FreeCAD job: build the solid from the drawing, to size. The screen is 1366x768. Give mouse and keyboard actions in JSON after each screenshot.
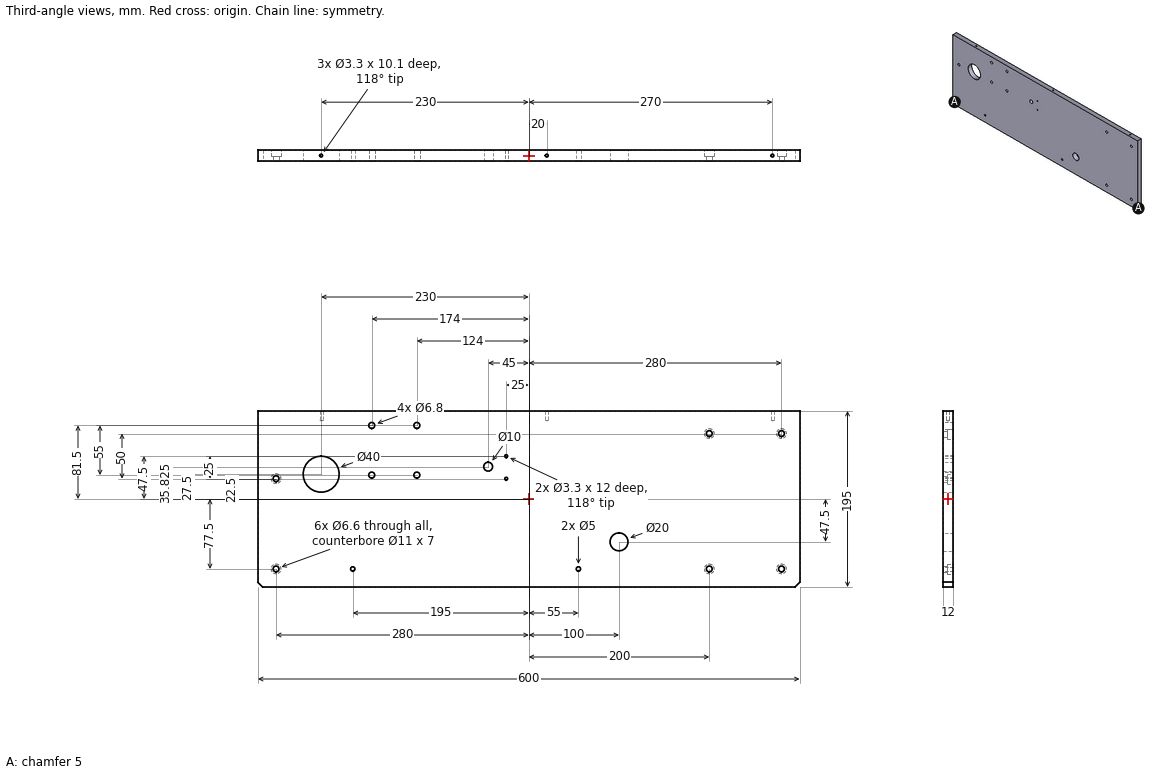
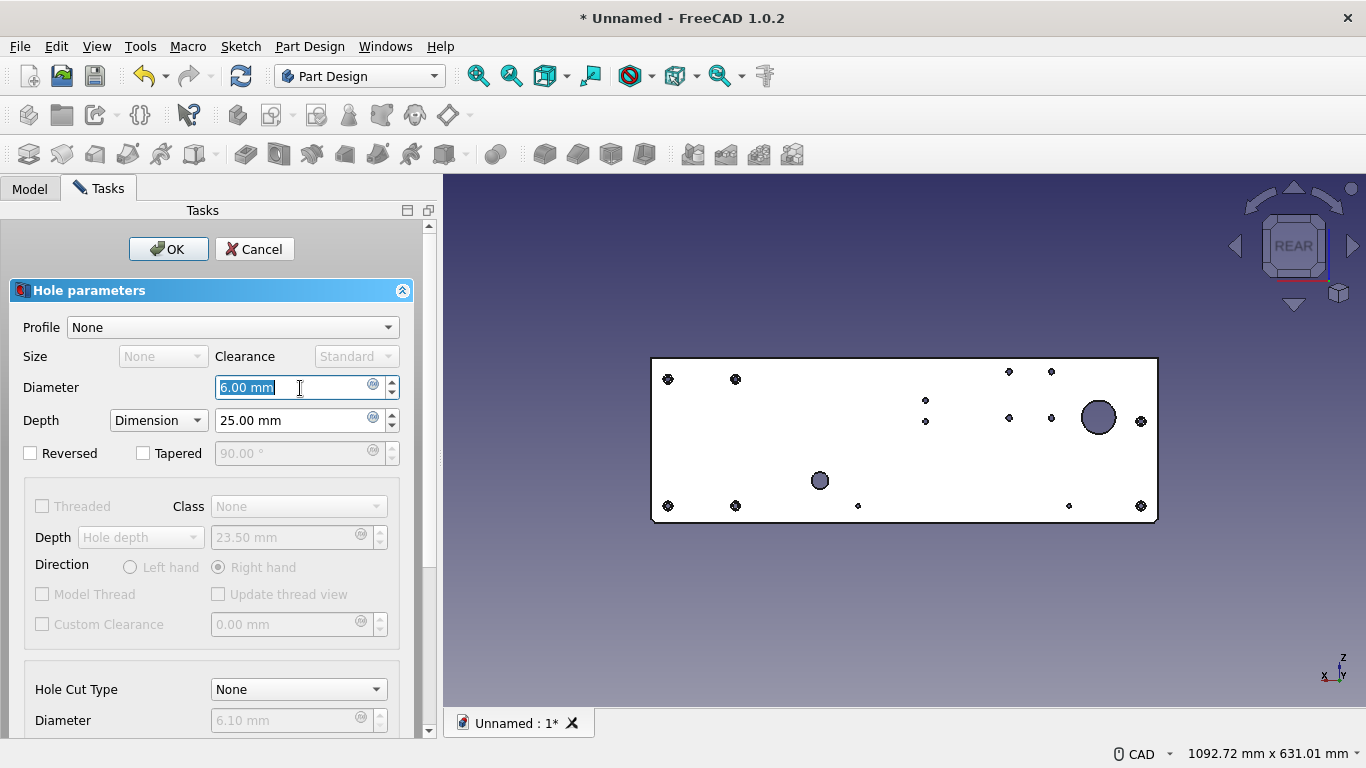
{"action": "type", "text": "3.3"}
{"action": "key", "text": "Tab"}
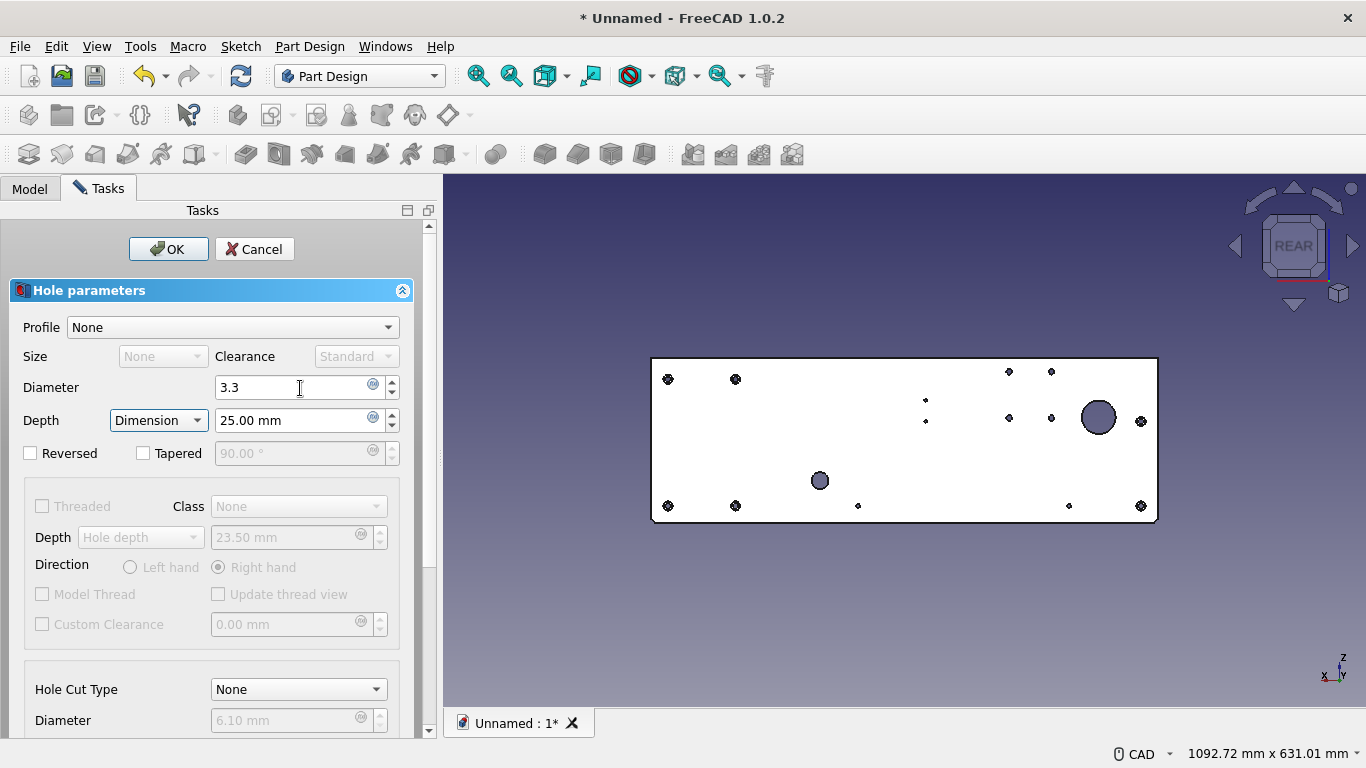
{"action": "triple_click", "coordinate": [300, 420]}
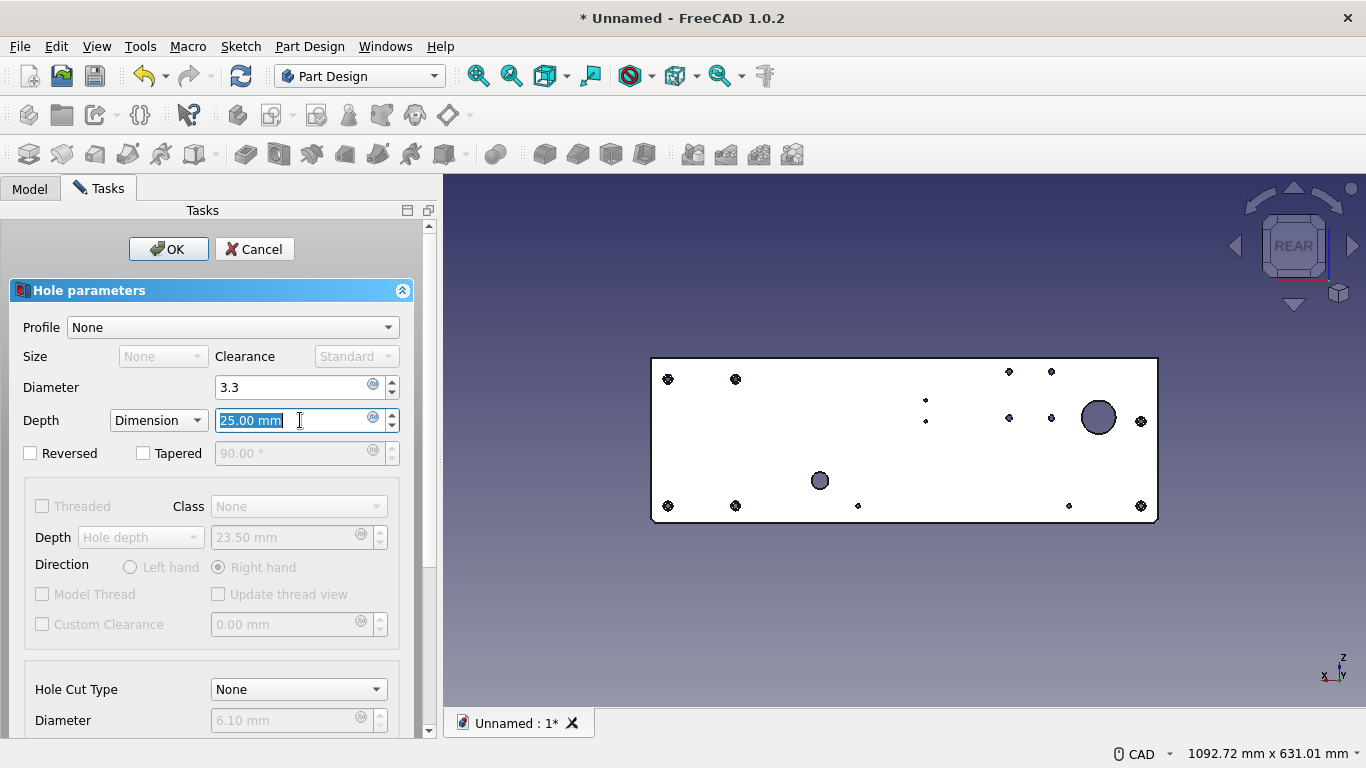
{"action": "type", "text": "12"}
{"action": "key", "text": "Tab"}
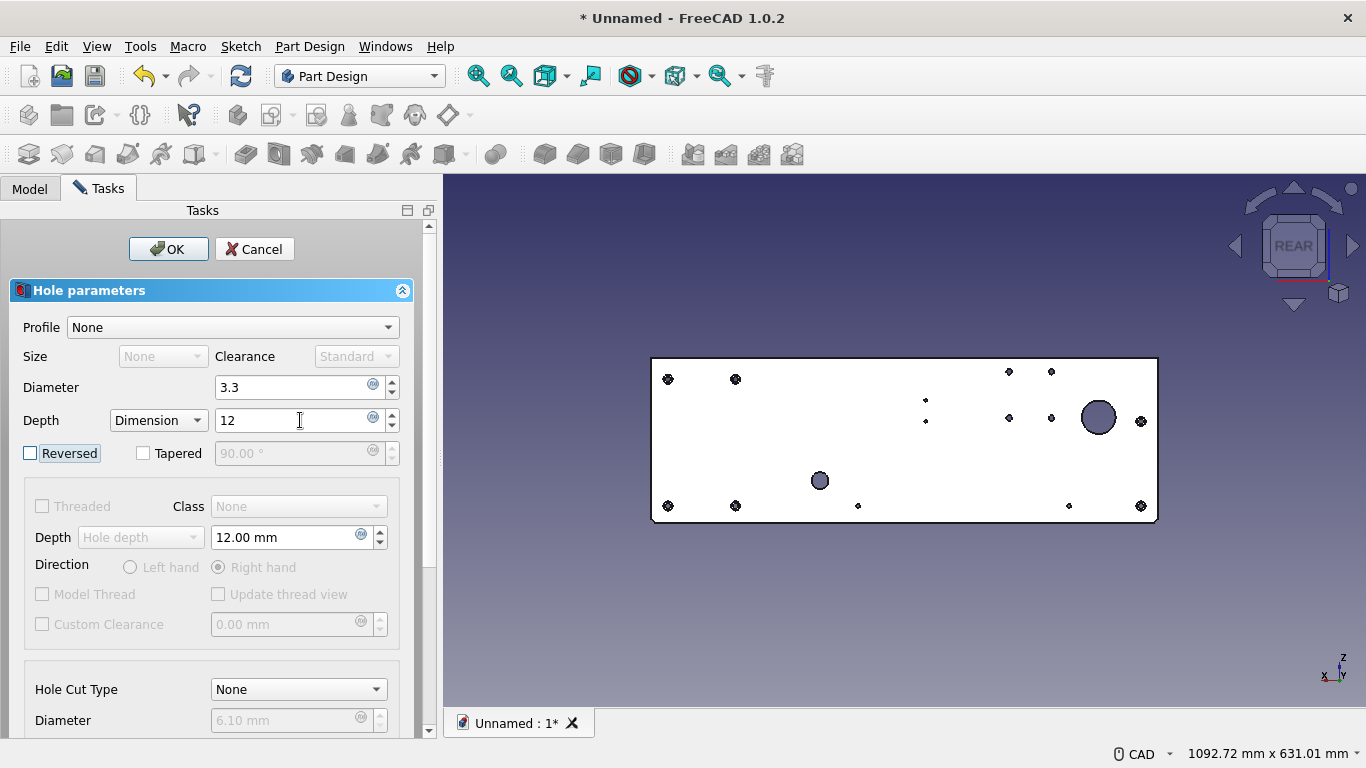
{"action": "left_click", "coordinate": [169, 249]}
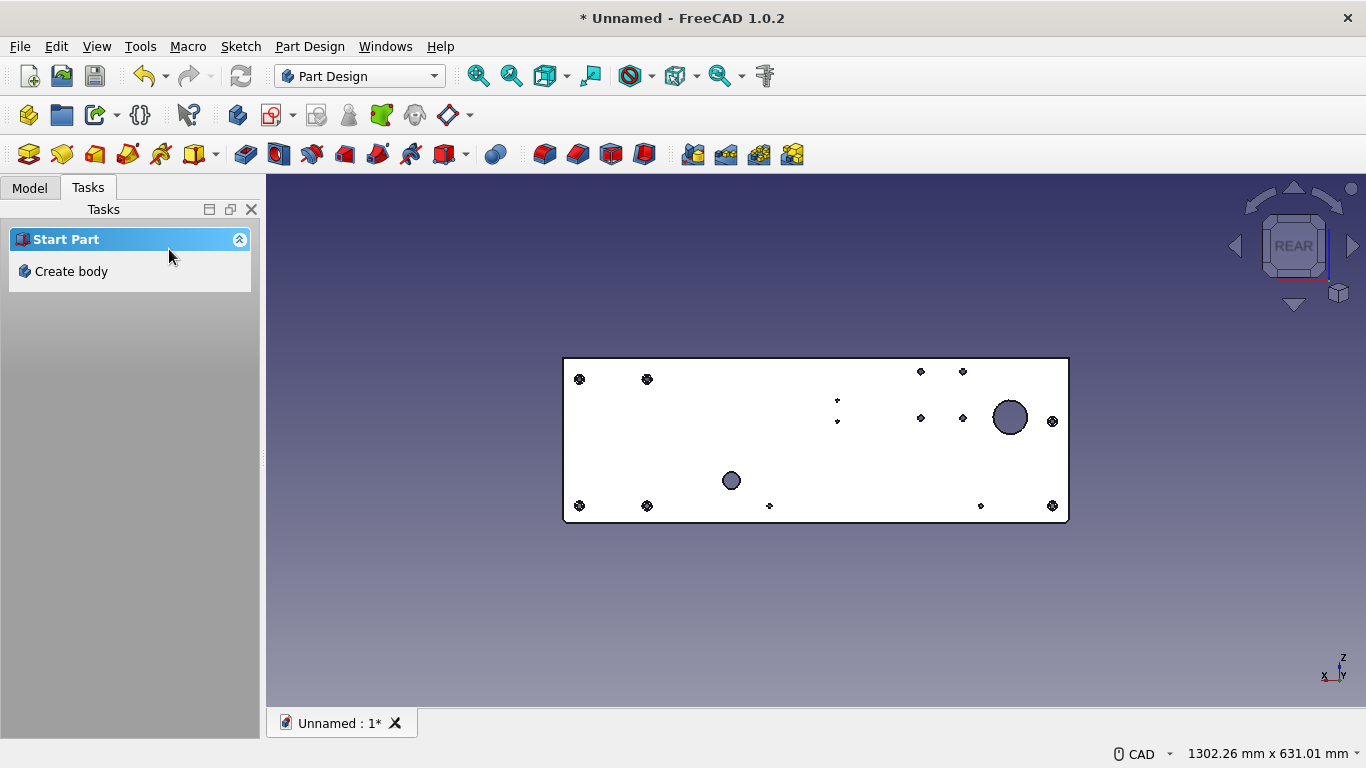
{"action": "left_click", "coordinate": [671, 439]}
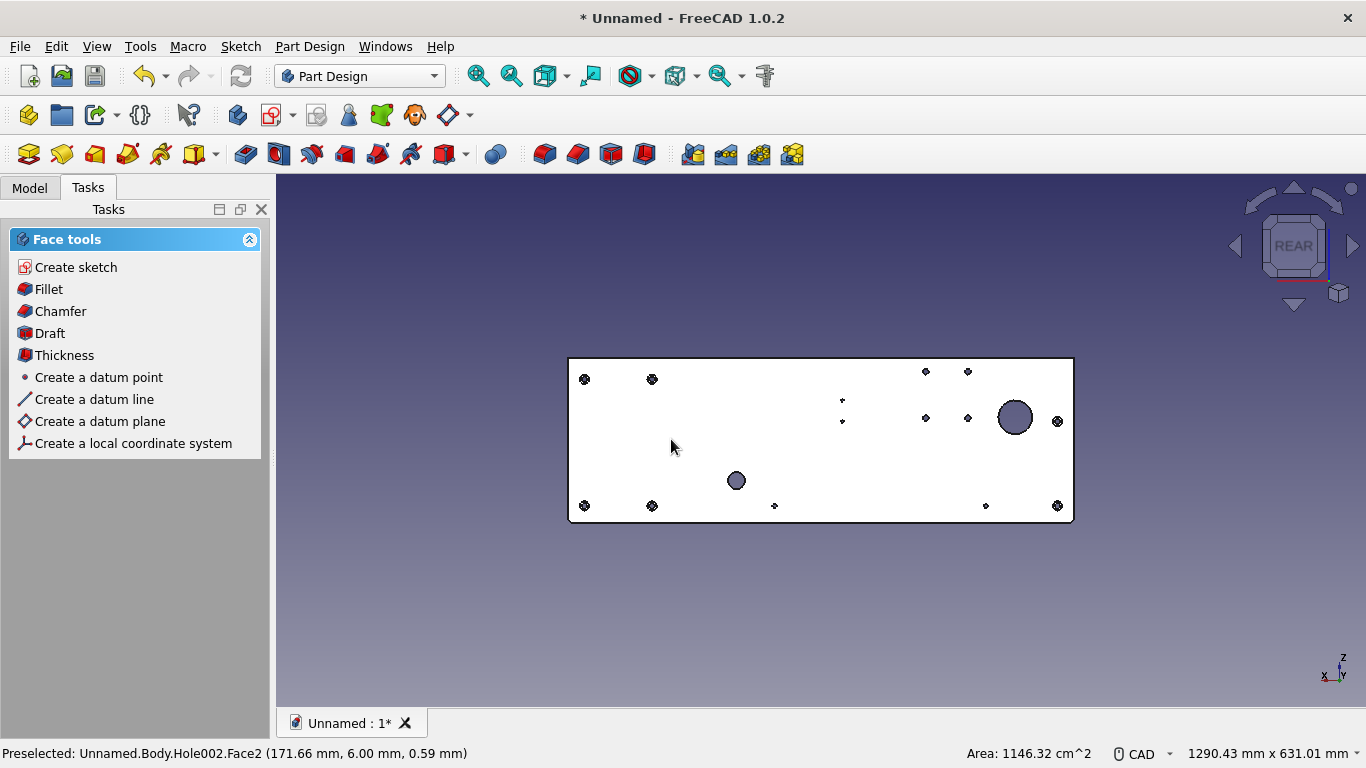
{"action": "left_click", "coordinate": [270, 116]}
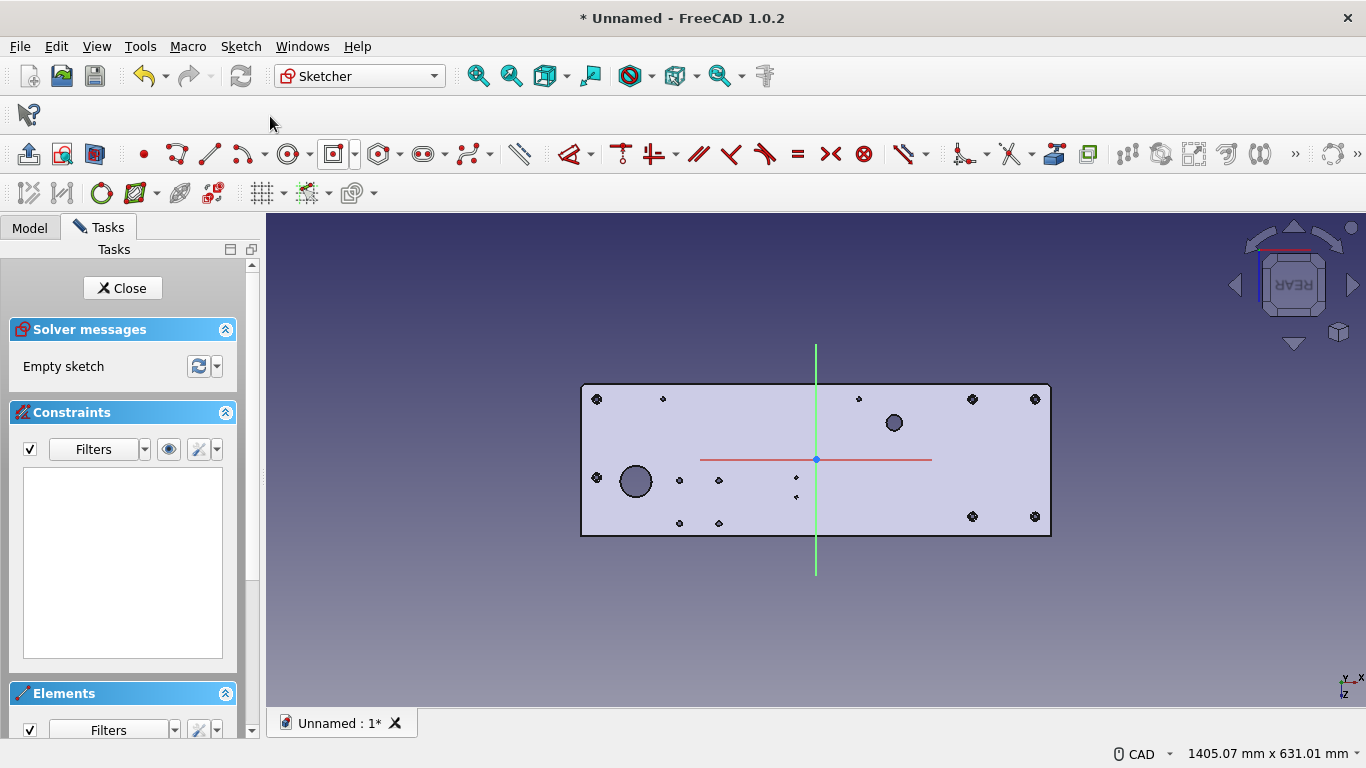
{"action": "scroll", "coordinate": [783, 490], "scroll_direction": "up", "scroll_amount": 15}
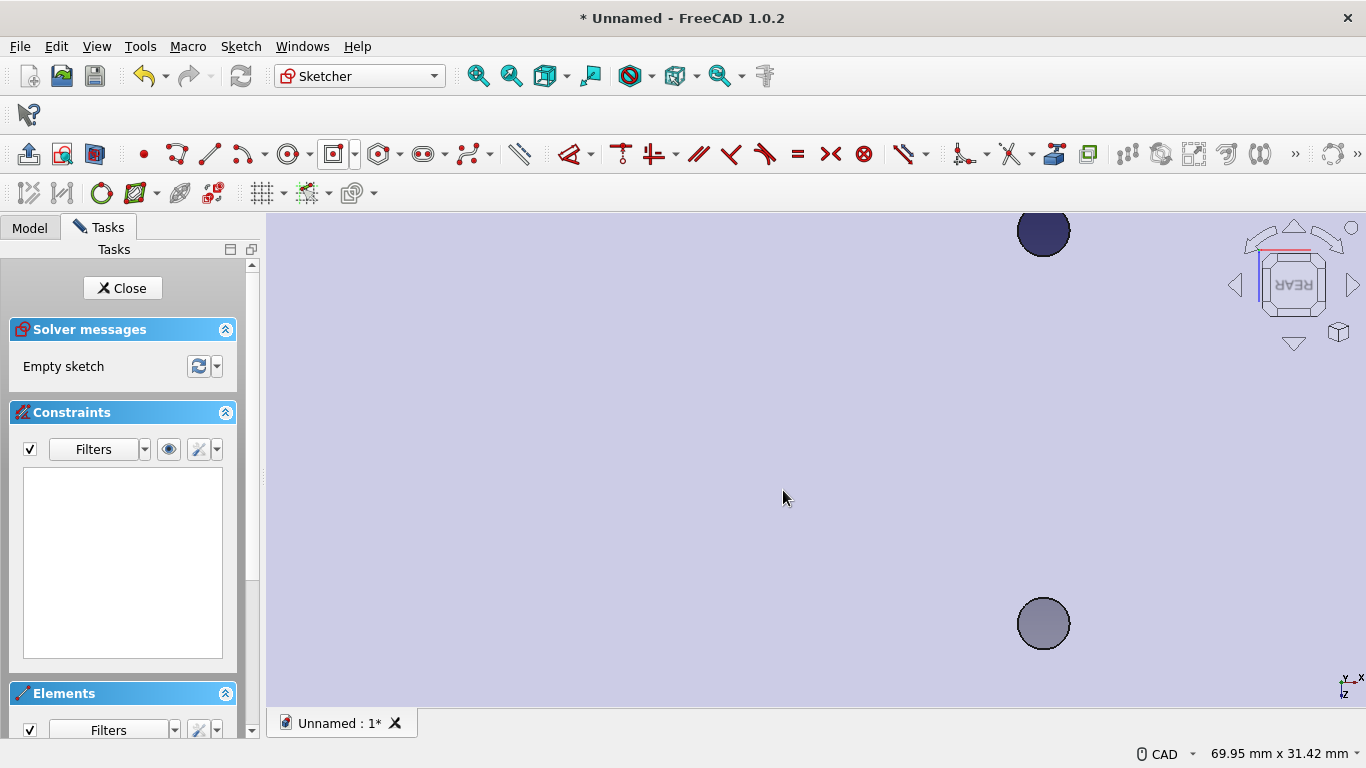
{"action": "scroll", "coordinate": [707, 416], "scroll_direction": "up", "scroll_amount": 3}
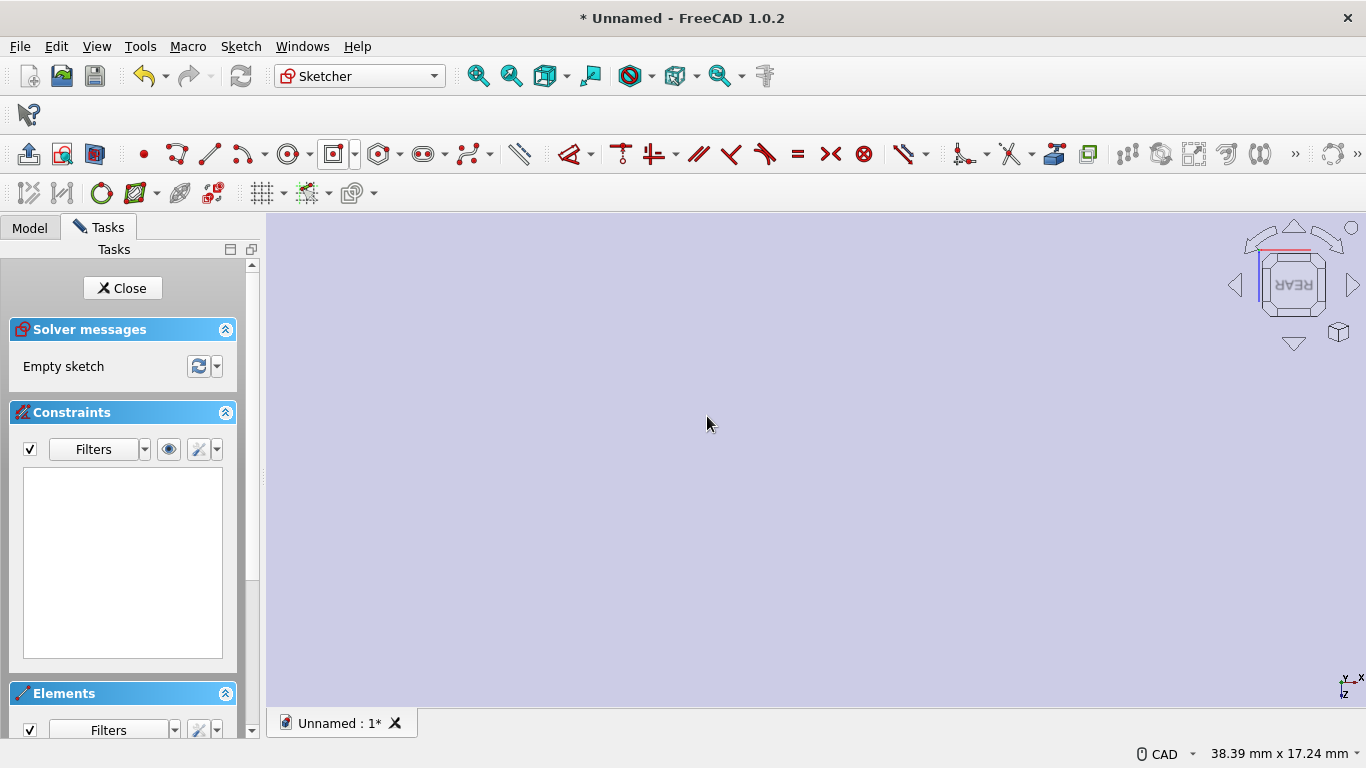
{"action": "key", "text": "g c"}